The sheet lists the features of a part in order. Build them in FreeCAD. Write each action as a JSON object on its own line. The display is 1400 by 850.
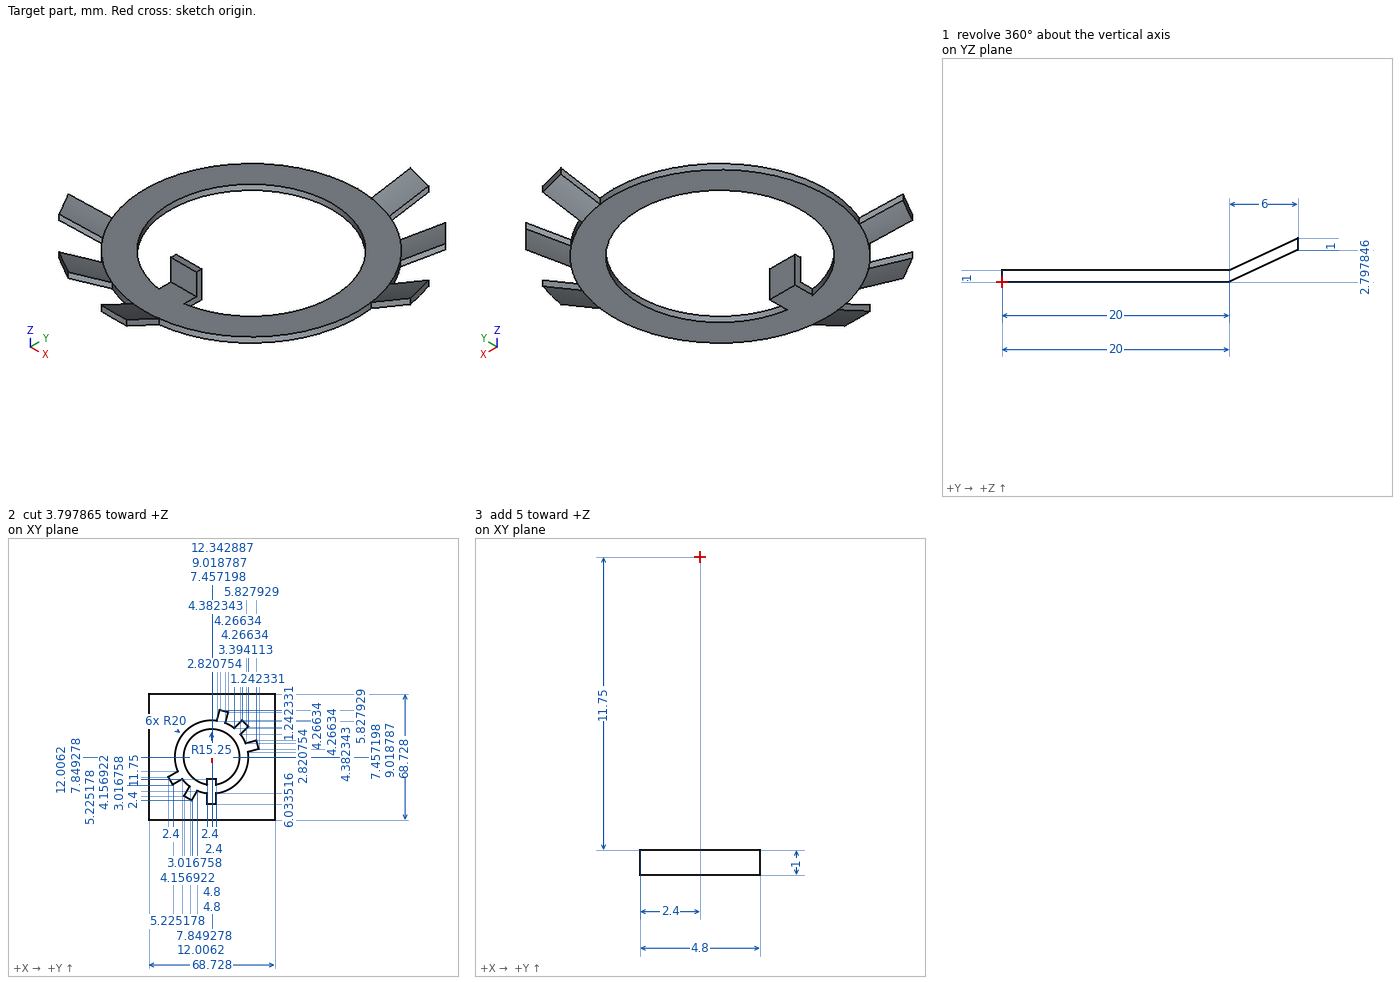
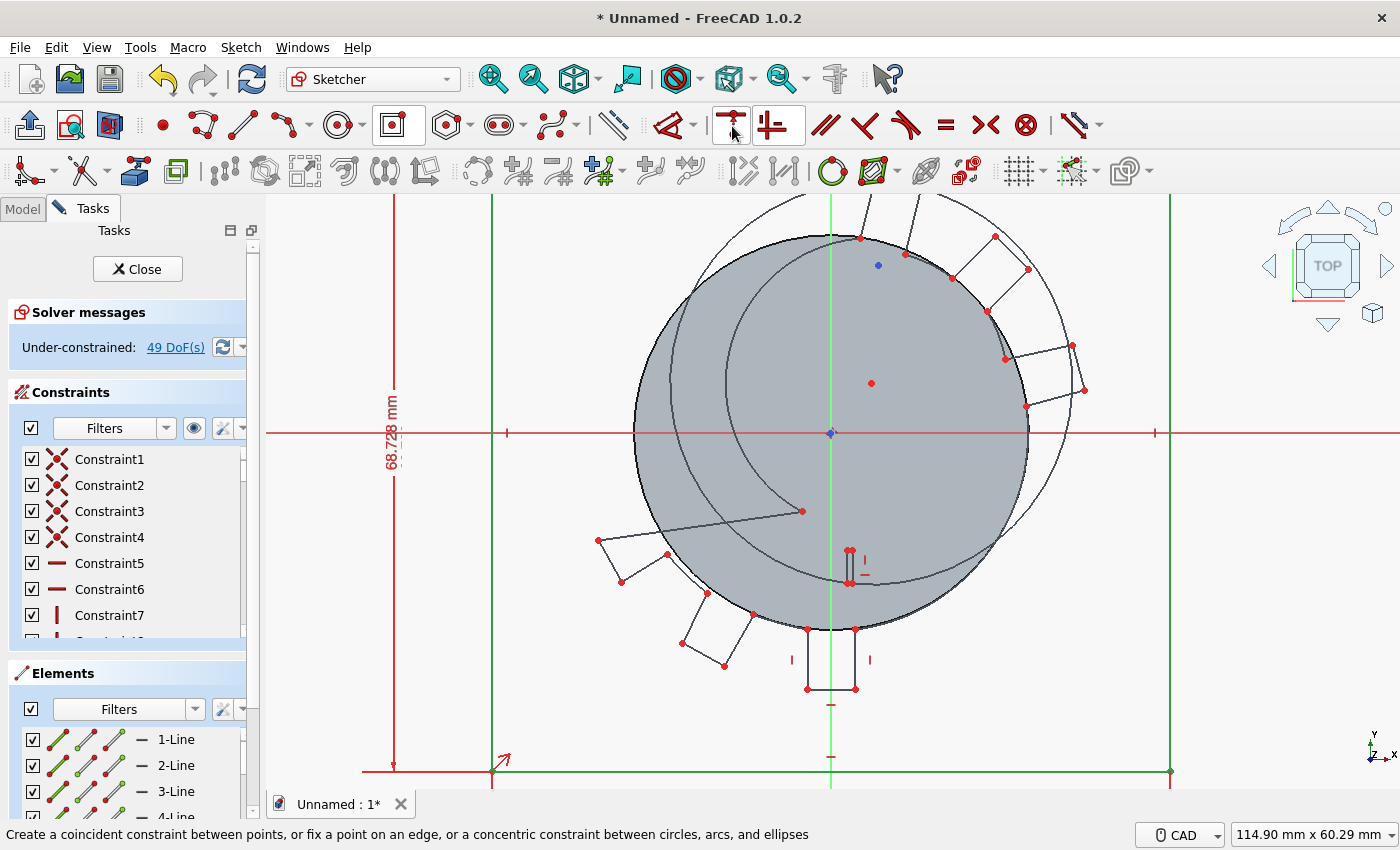
{"action": "left_click", "coordinate": [688, 301]}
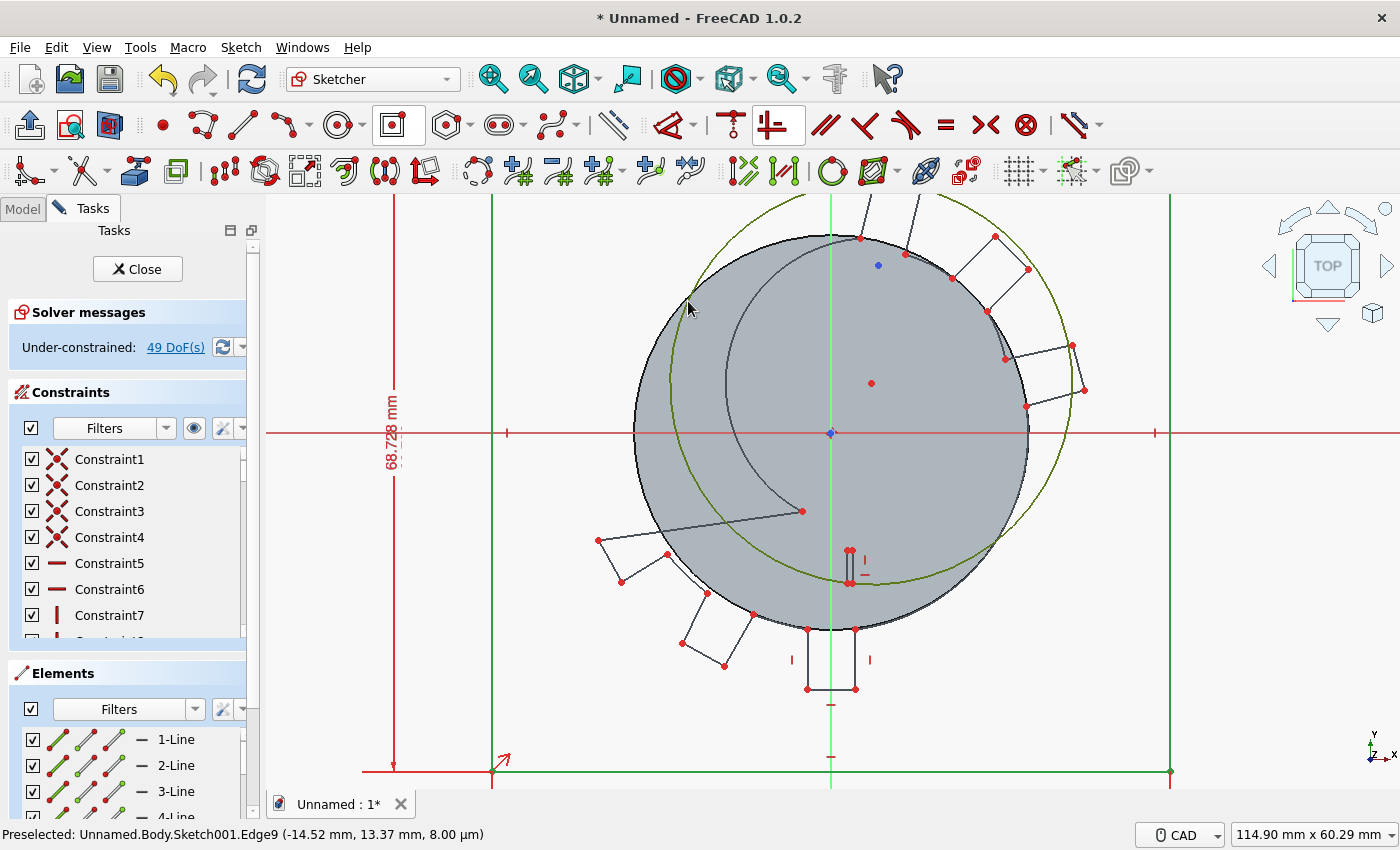
{"action": "left_click", "coordinate": [942, 597]}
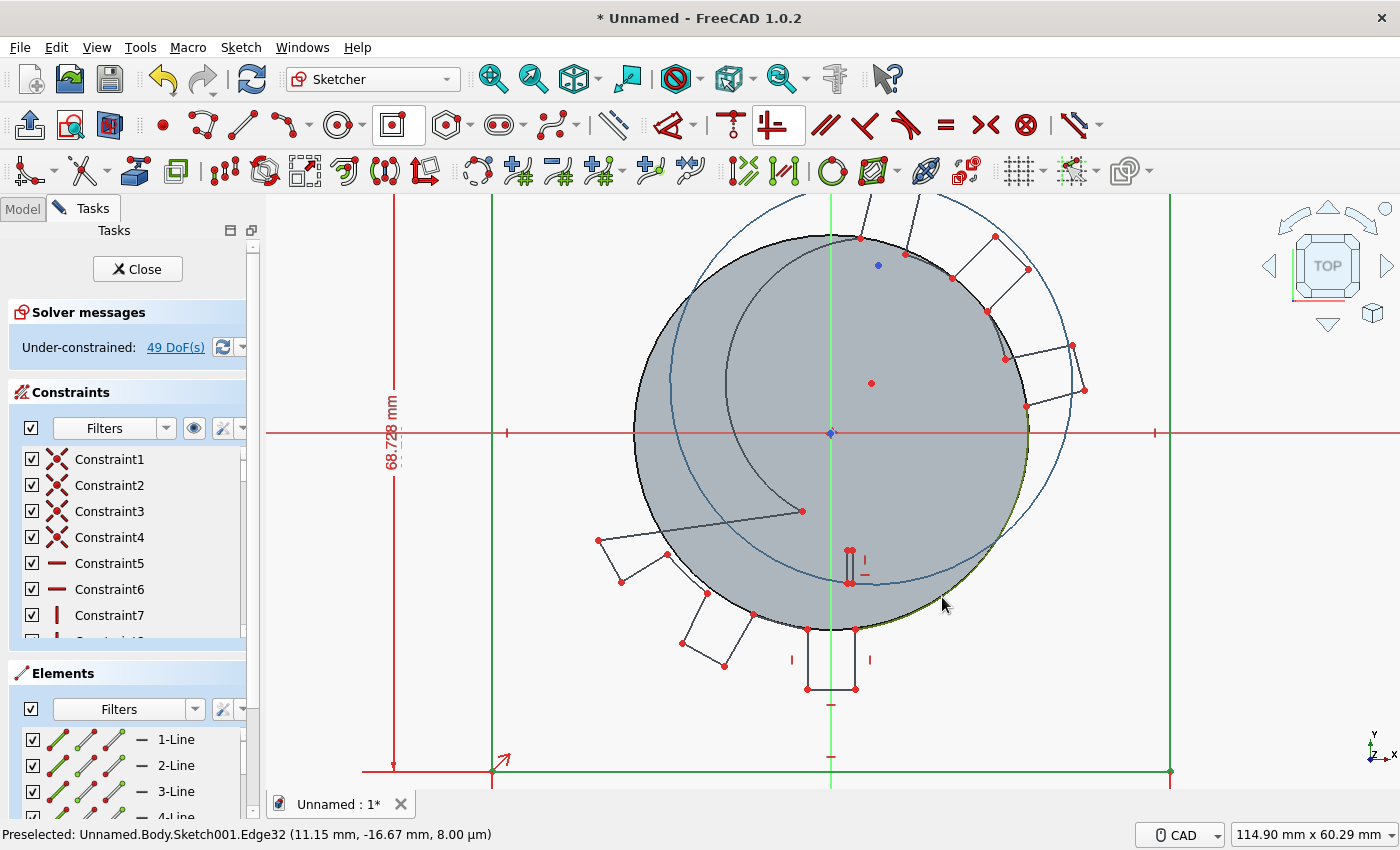
{"action": "left_click", "coordinate": [732, 126]}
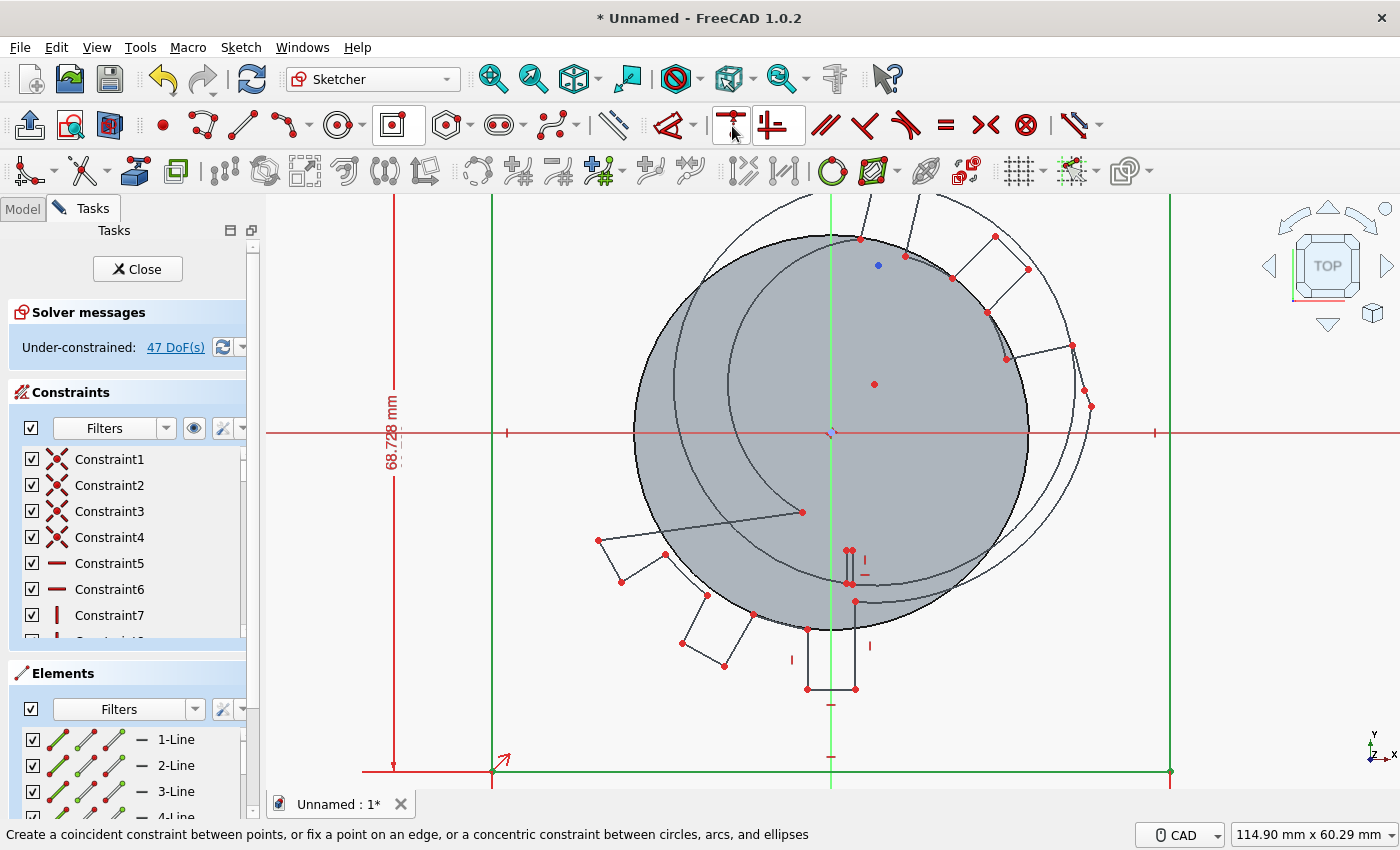
{"action": "left_click", "coordinate": [693, 299]}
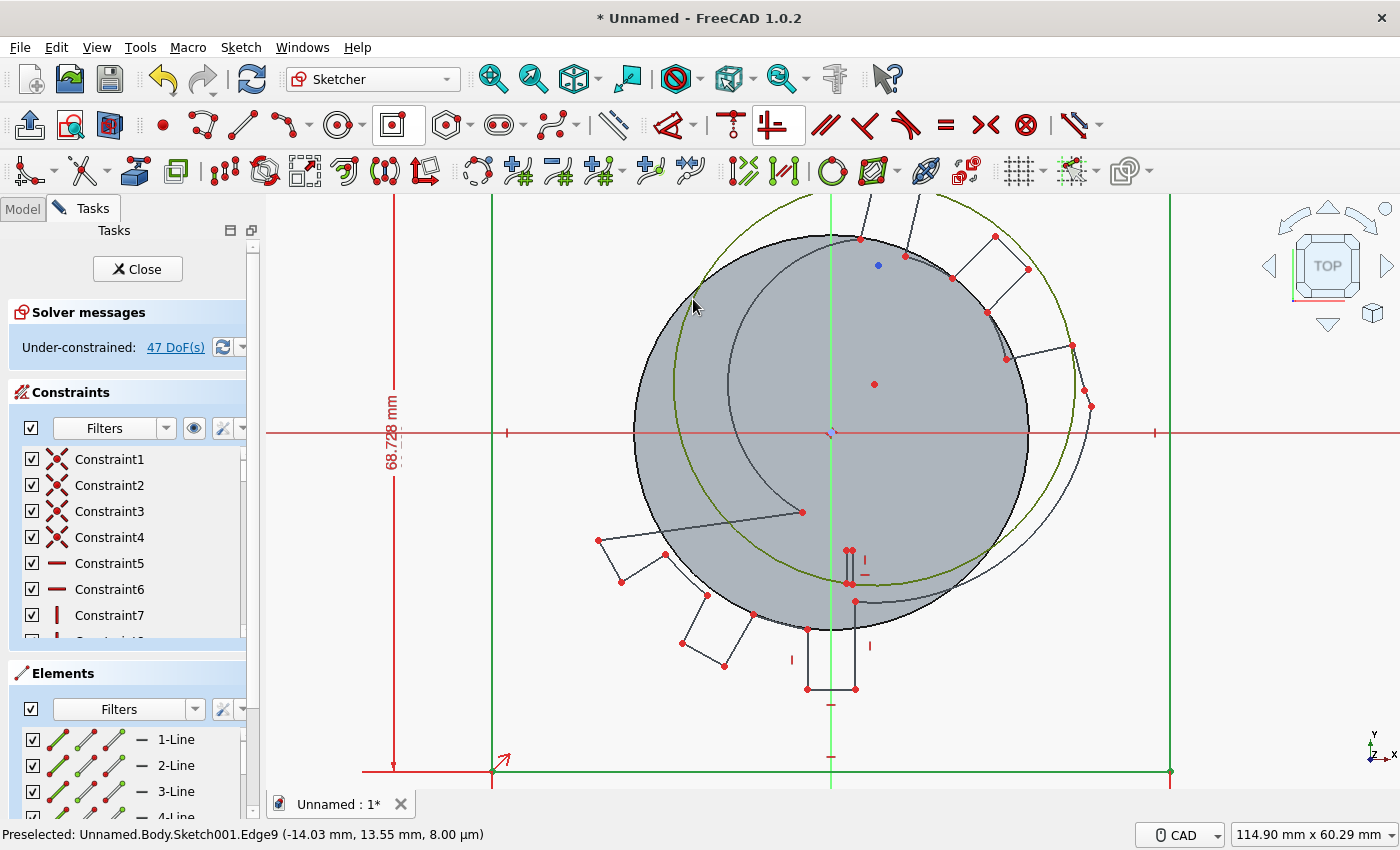
{"action": "left_click", "coordinate": [770, 620]}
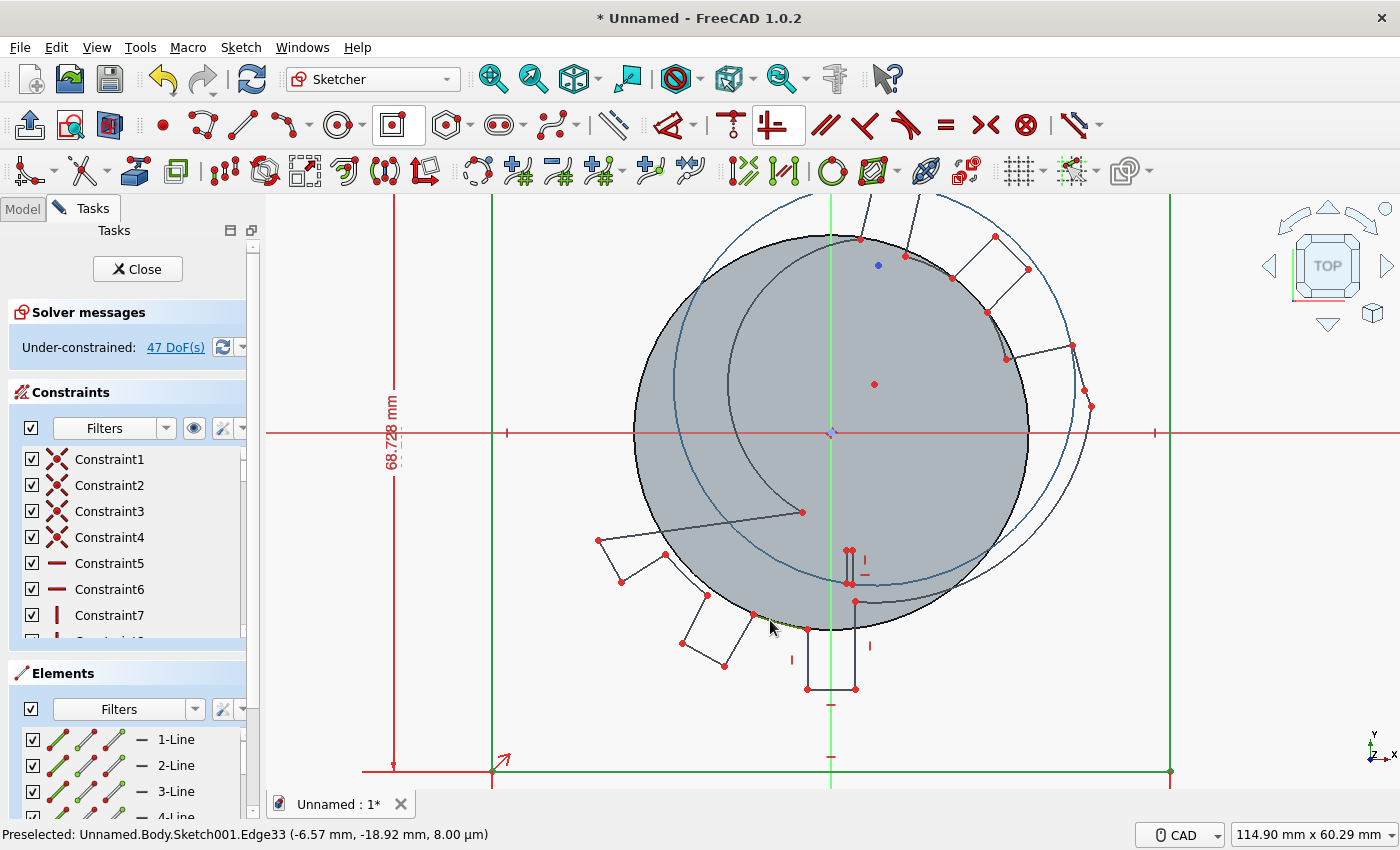
{"action": "left_click", "coordinate": [732, 126]}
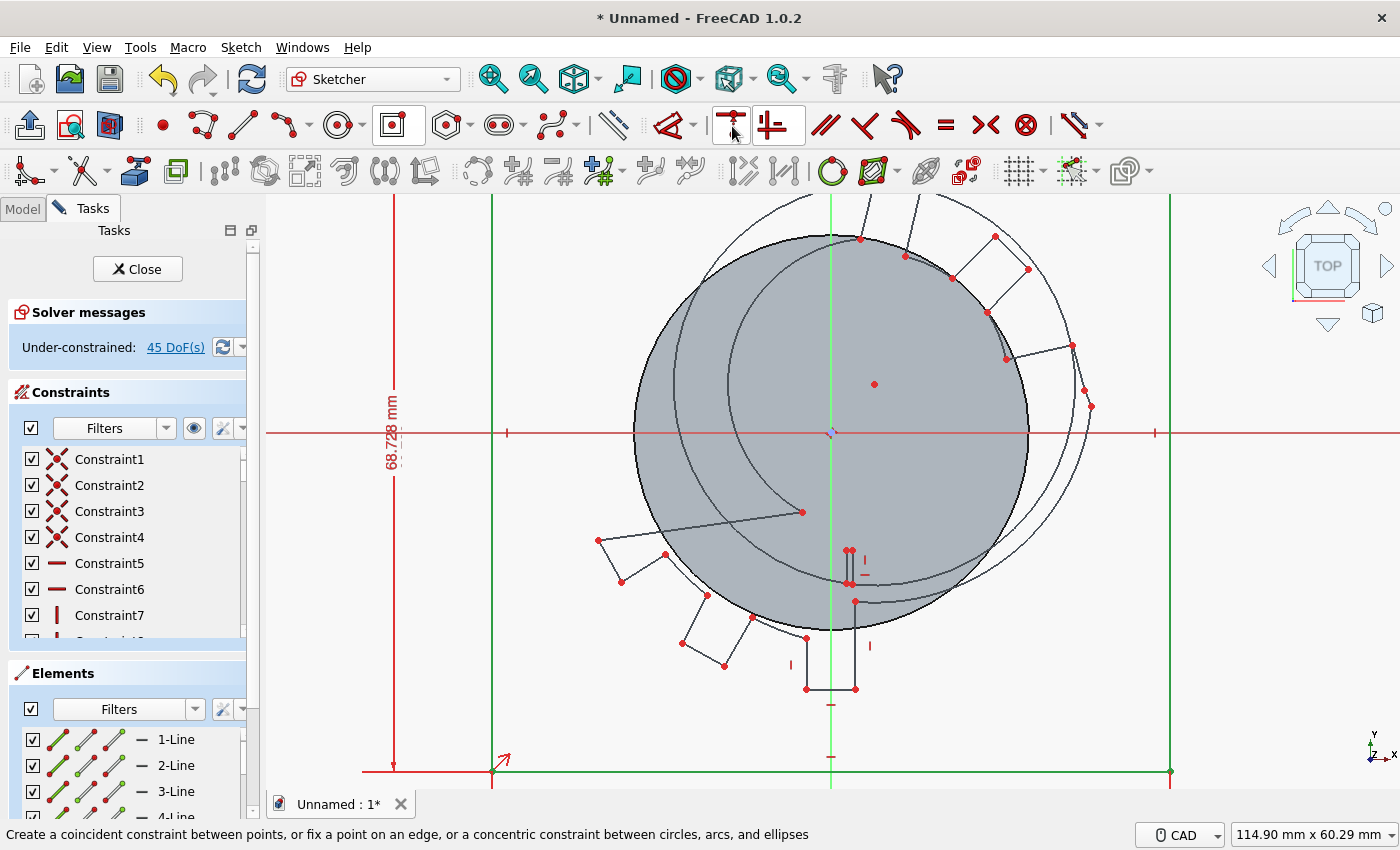
{"action": "left_click_drag", "start_coordinate": [821, 375], "coordinate": [884, 443]}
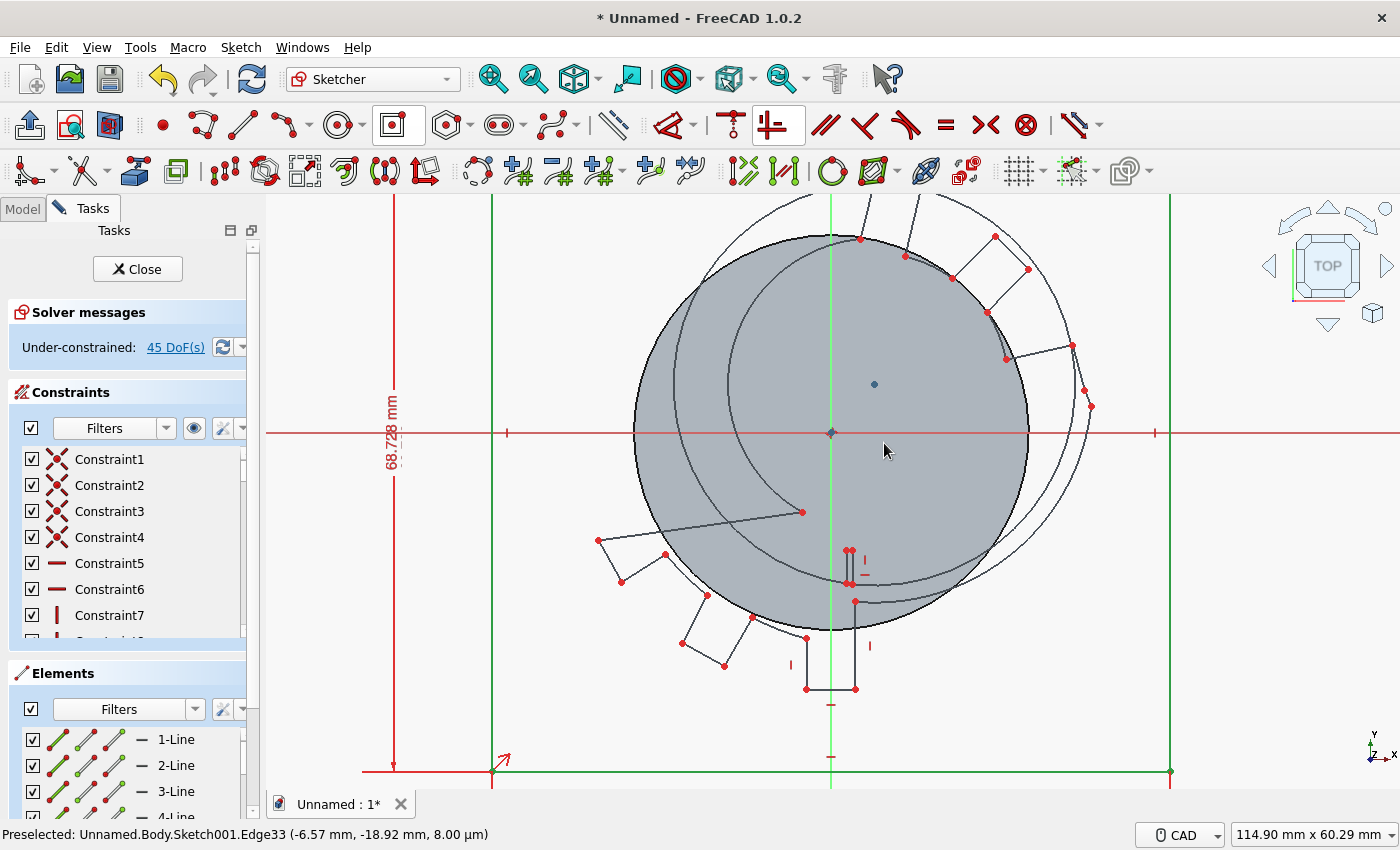
{"action": "left_click", "coordinate": [732, 126]}